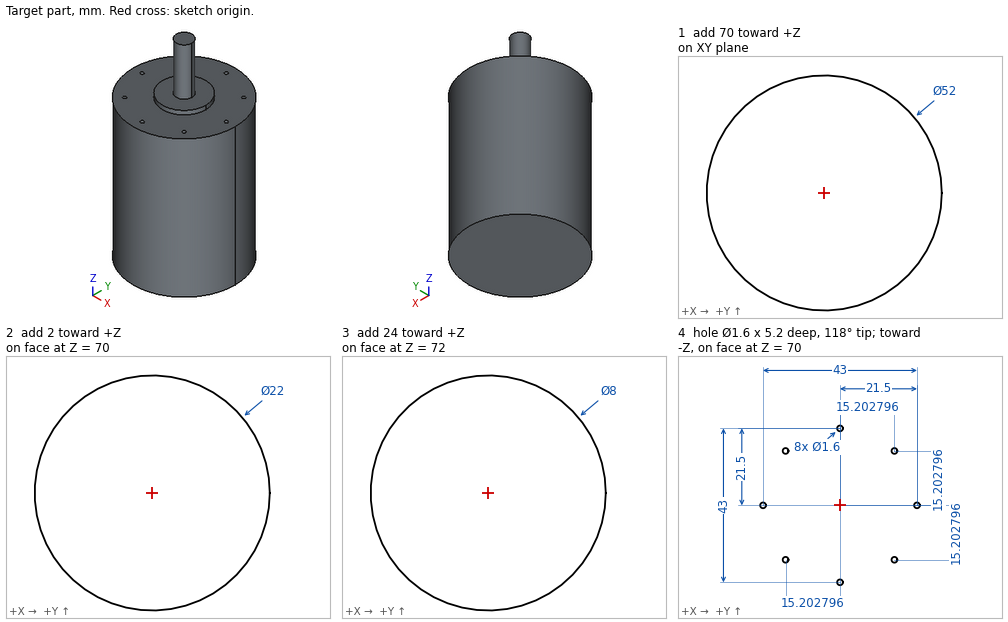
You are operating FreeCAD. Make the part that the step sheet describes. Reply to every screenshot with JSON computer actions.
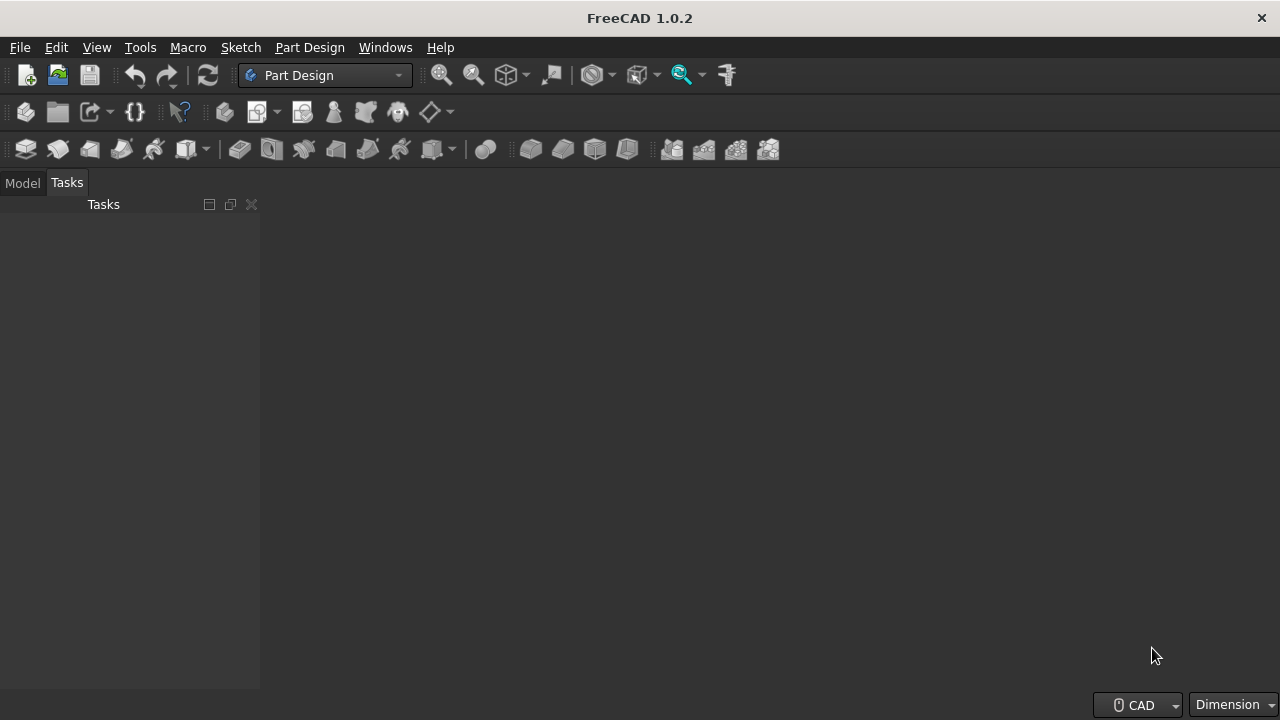
{"action": "left_click", "coordinate": [26, 76]}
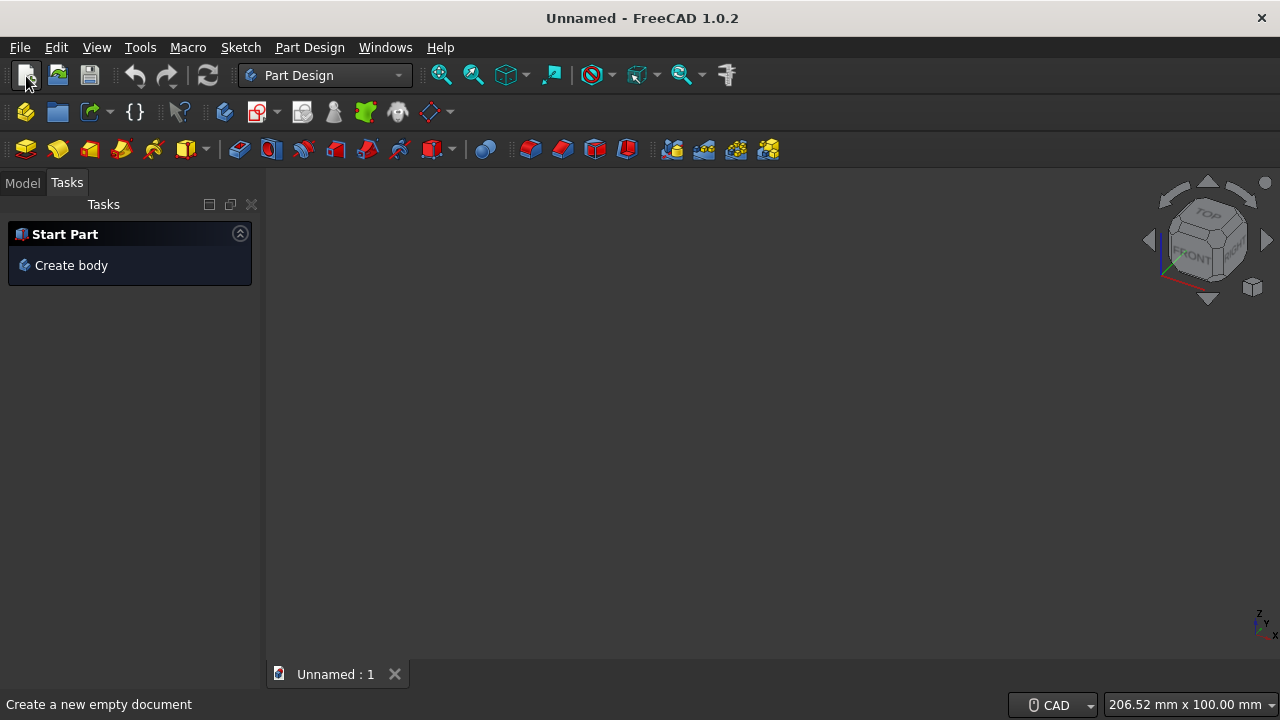
{"action": "left_click", "coordinate": [258, 112]}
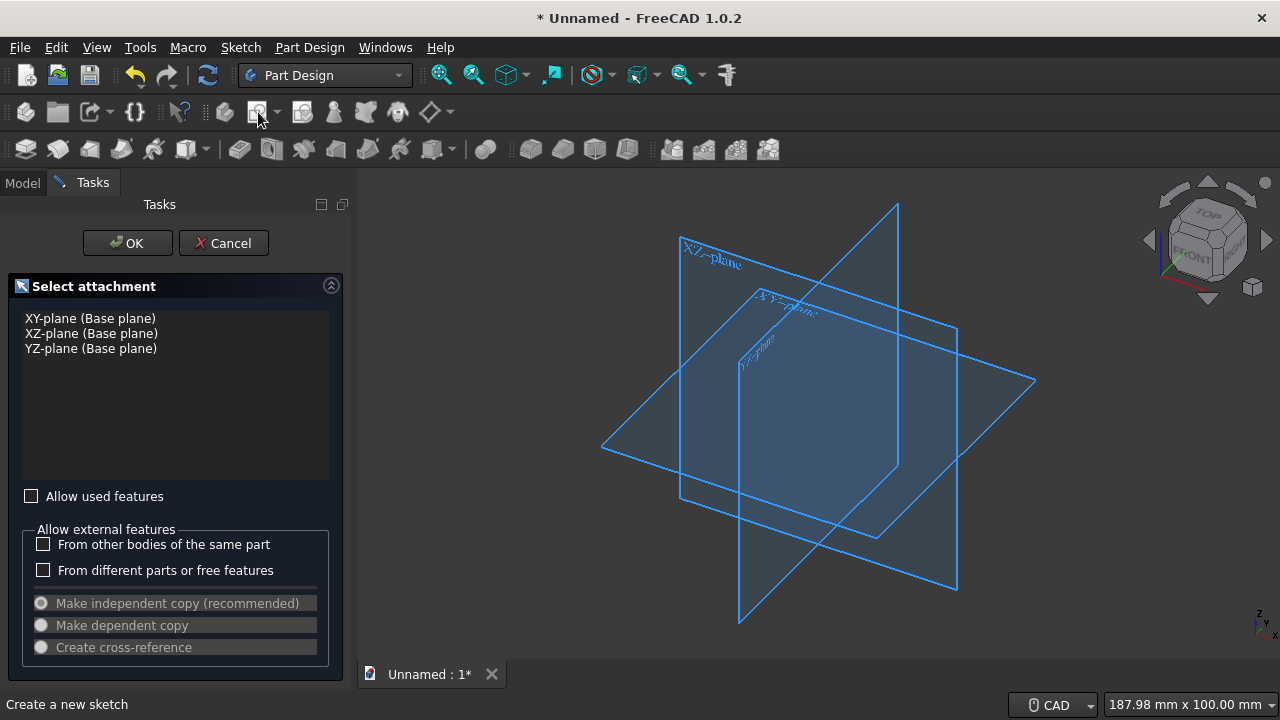
{"action": "left_click", "coordinate": [82, 318]}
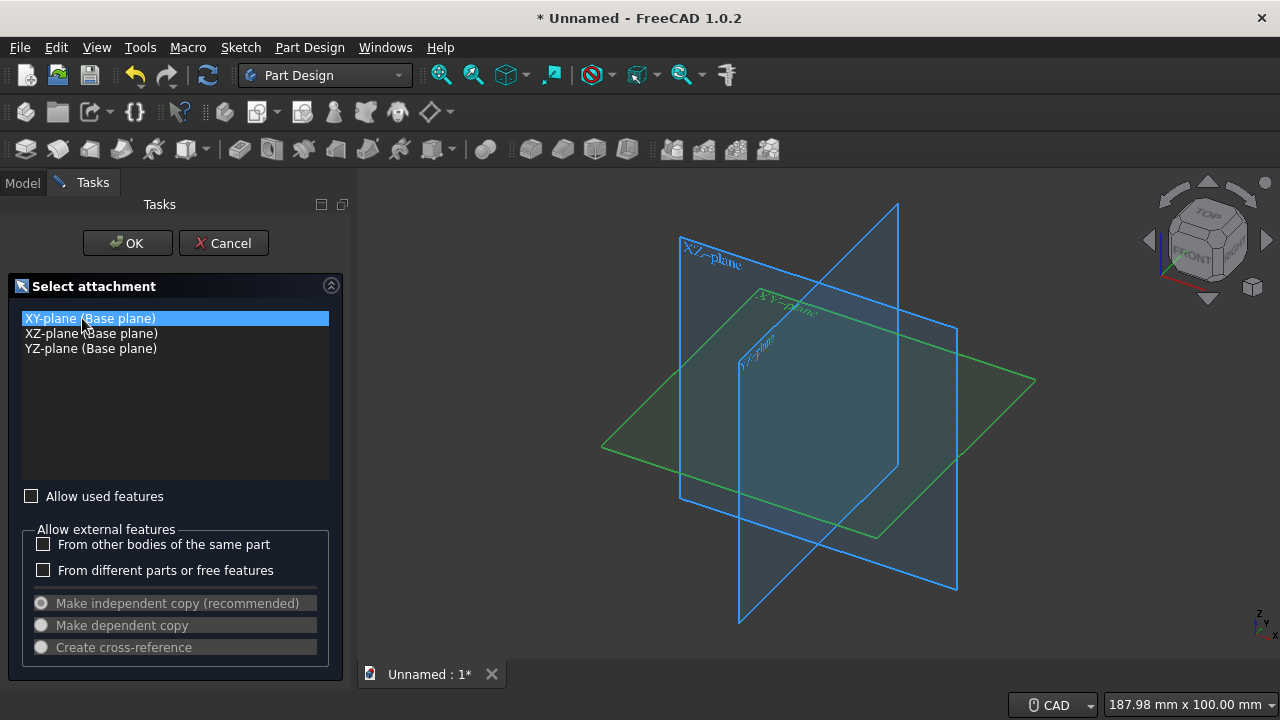
{"action": "left_click", "coordinate": [128, 243]}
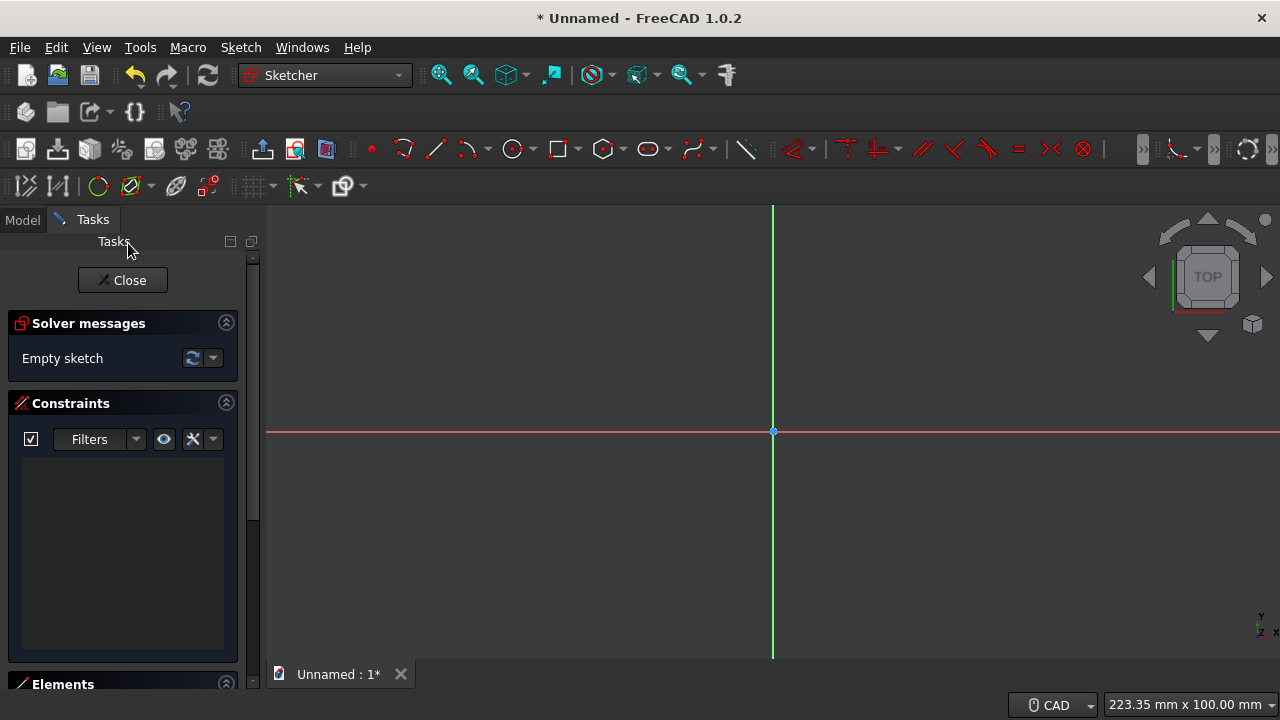
{"action": "left_click", "coordinate": [514, 150]}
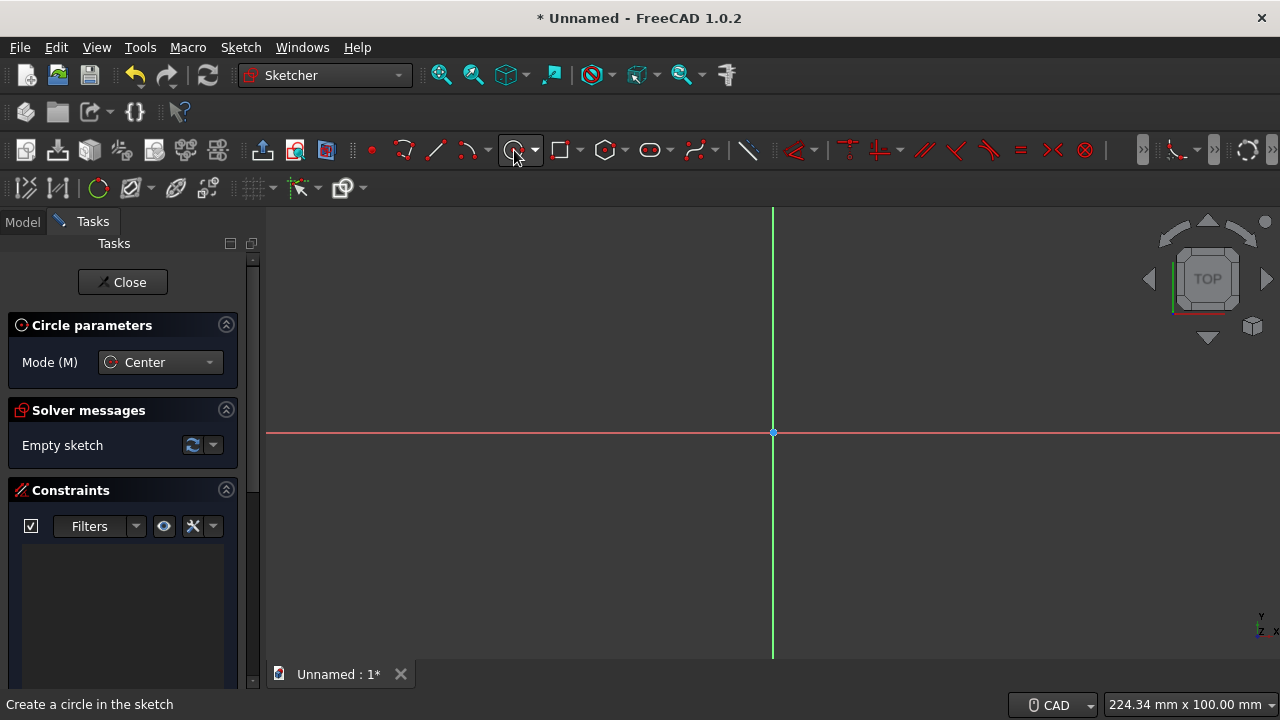
{"action": "left_click", "coordinate": [773, 433]}
{"action": "mouse_move", "coordinate": [856, 350]}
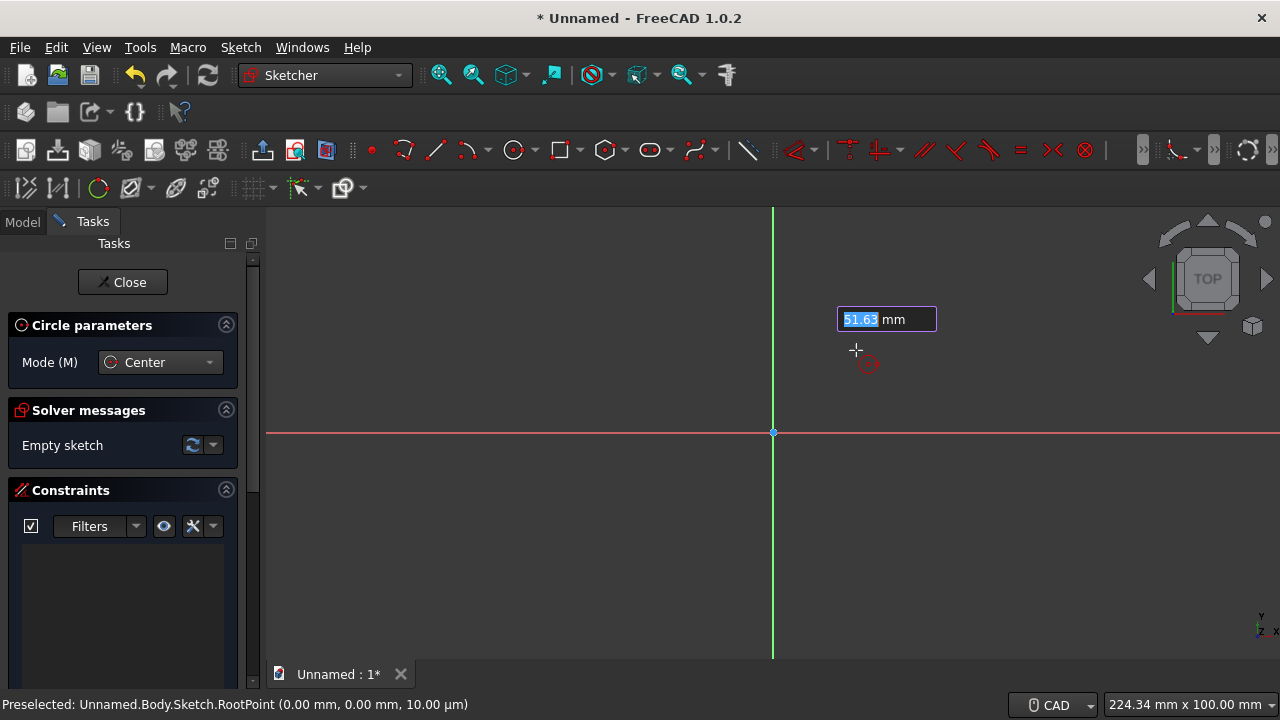
{"action": "type", "text": "52"}
{"action": "key", "text": "Return"}
{"action": "key", "text": "Escape"}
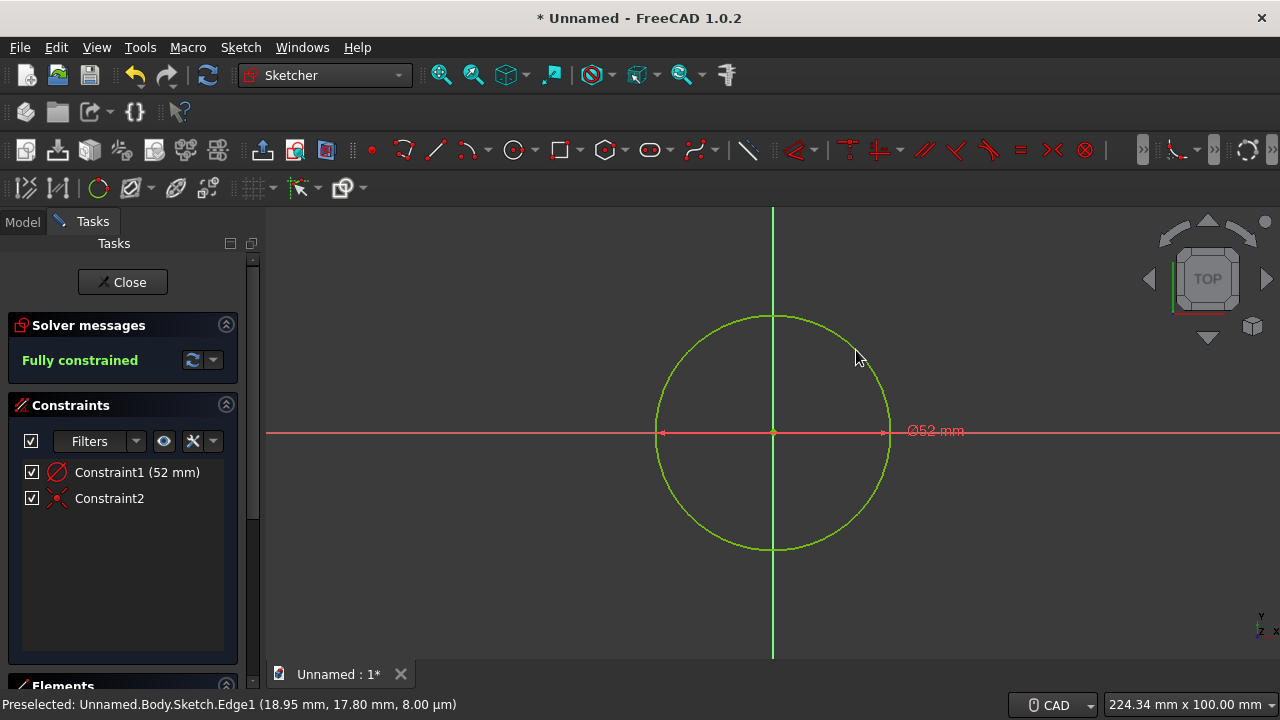
{"action": "left_click", "coordinate": [123, 282]}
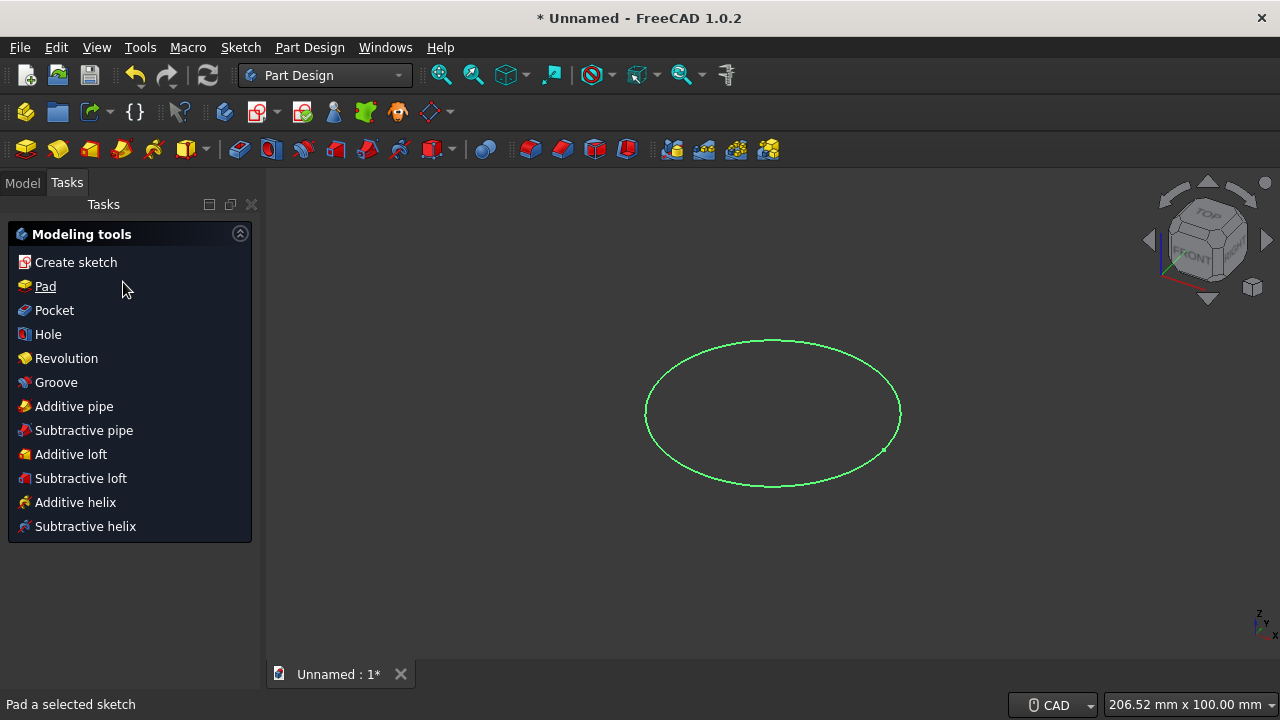
{"action": "left_click", "coordinate": [26, 150]}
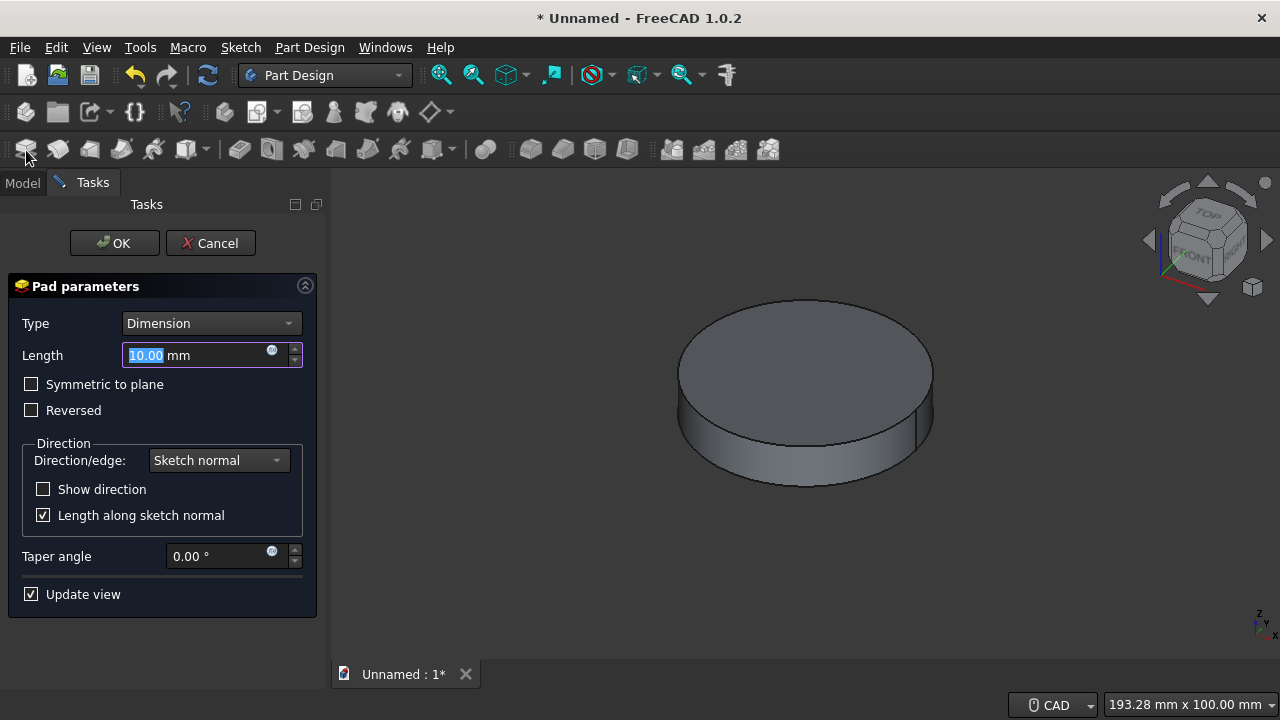
{"action": "type", "text": "70"}
{"action": "key", "text": "Tab"}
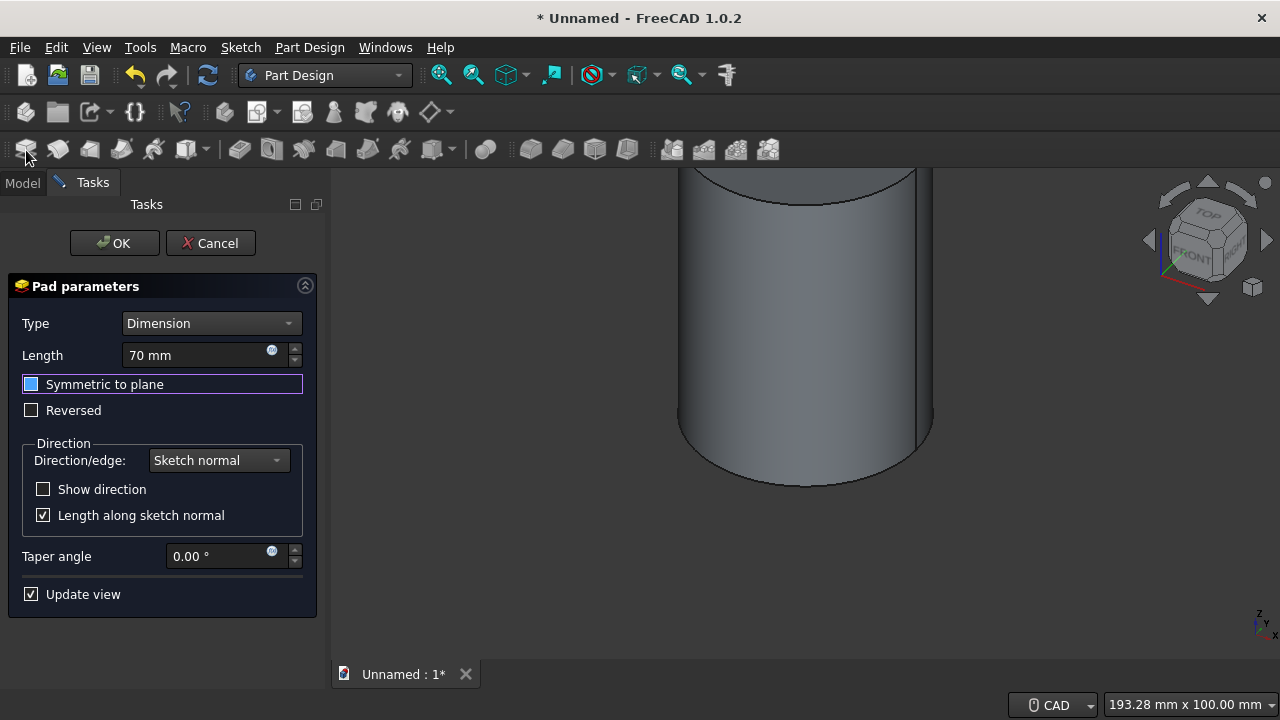
{"action": "left_click", "coordinate": [115, 243]}